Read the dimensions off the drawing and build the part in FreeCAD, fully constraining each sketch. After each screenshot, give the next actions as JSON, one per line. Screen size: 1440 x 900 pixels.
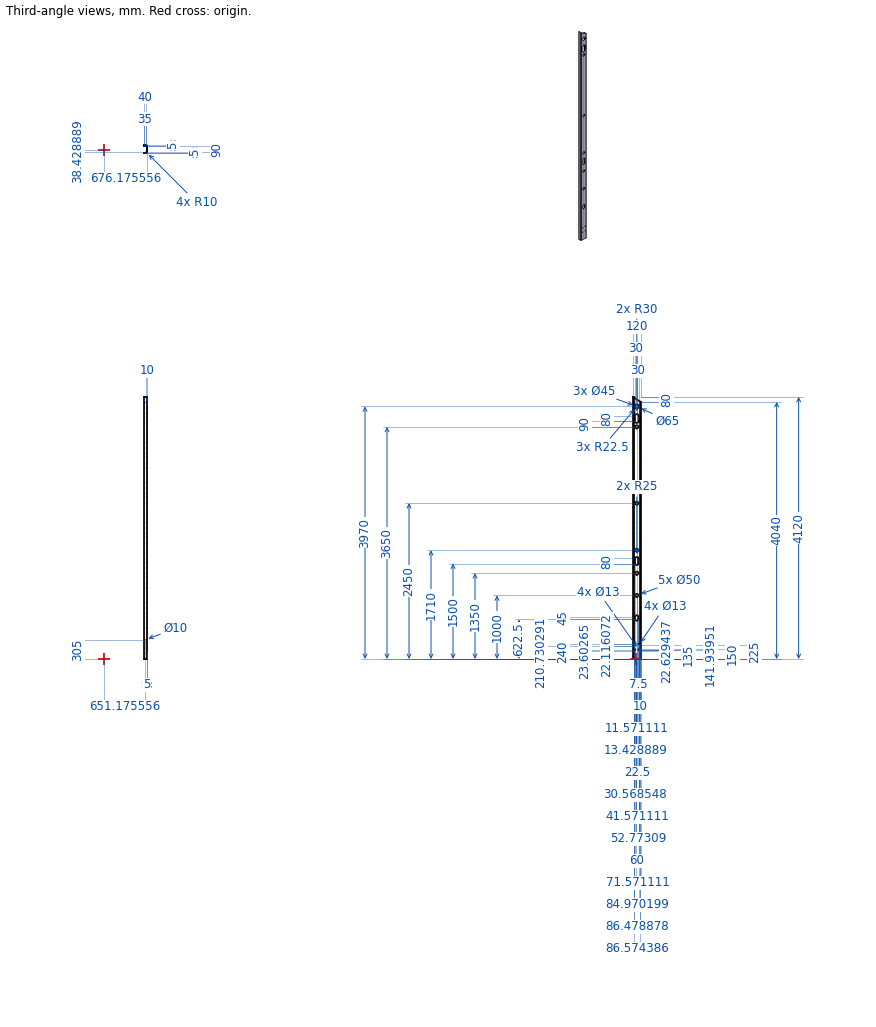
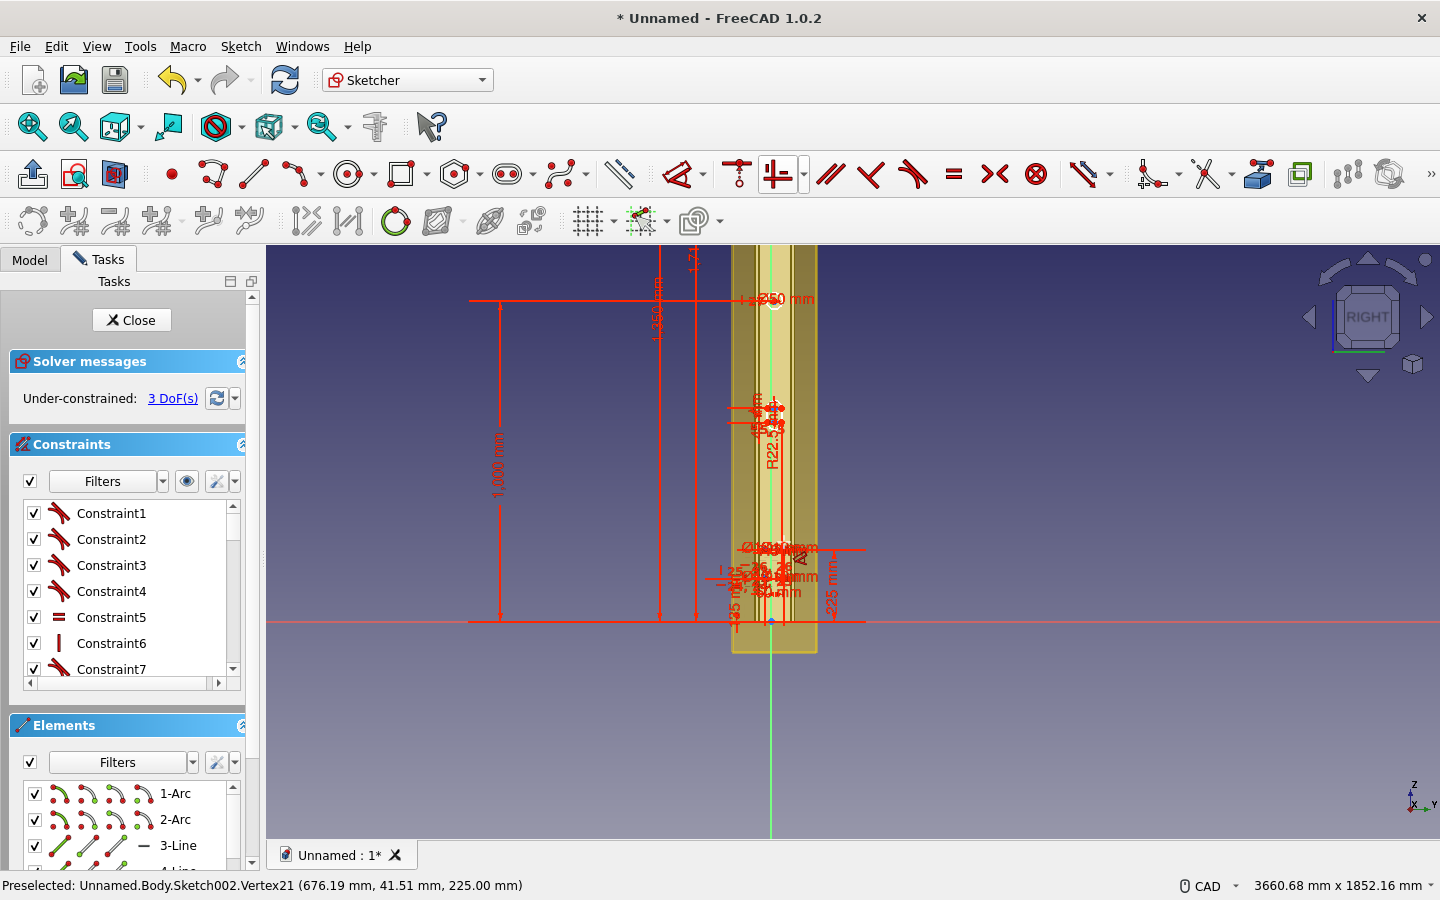
{"action": "scroll", "coordinate": [789, 784], "scroll_direction": "down", "scroll_amount": 6}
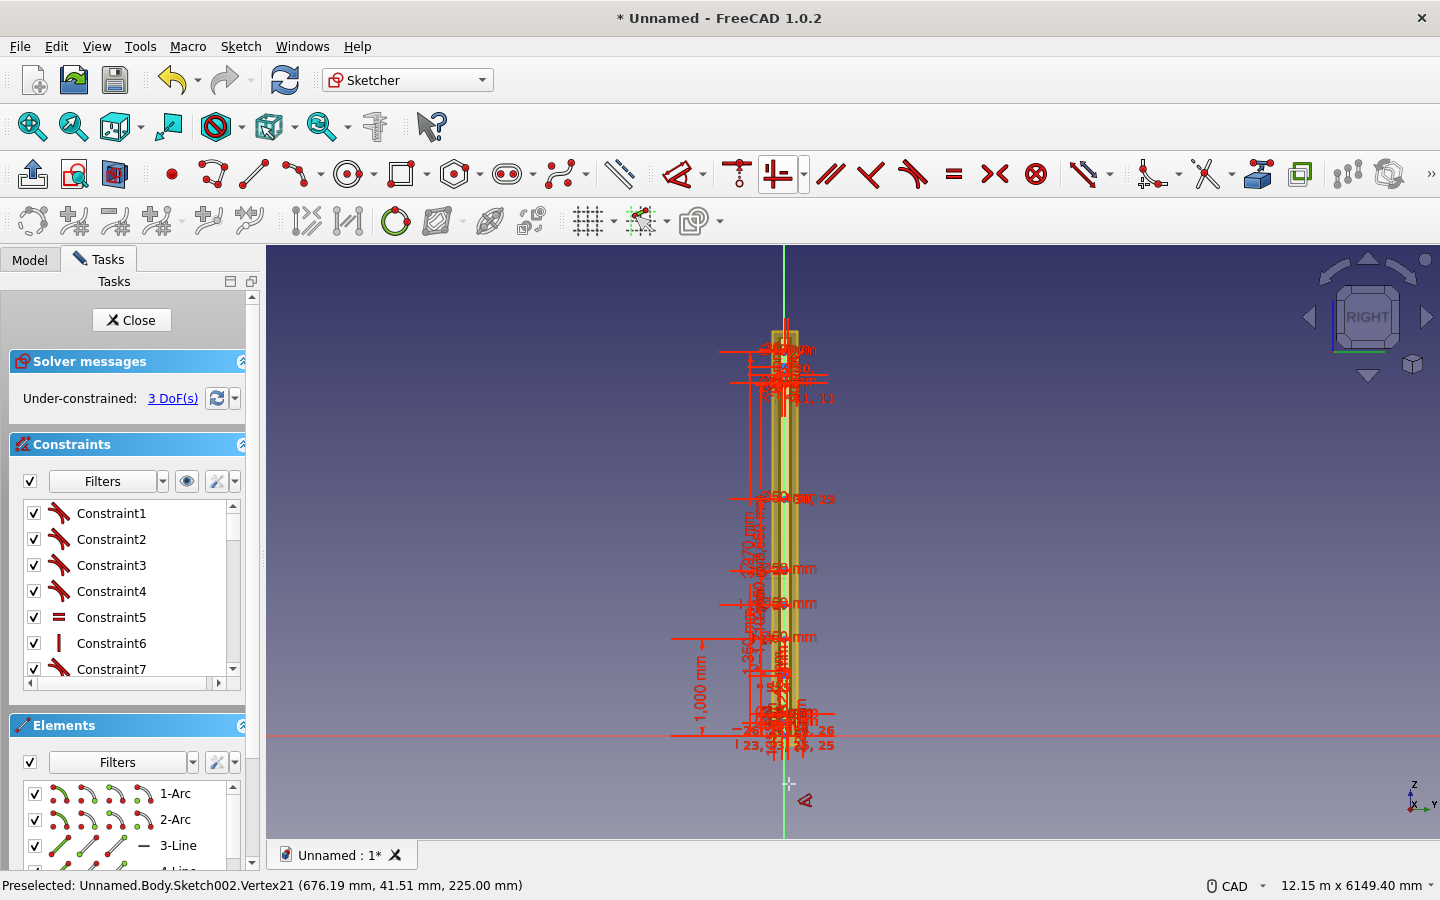
{"action": "scroll", "coordinate": [787, 671], "scroll_direction": "up", "scroll_amount": 15}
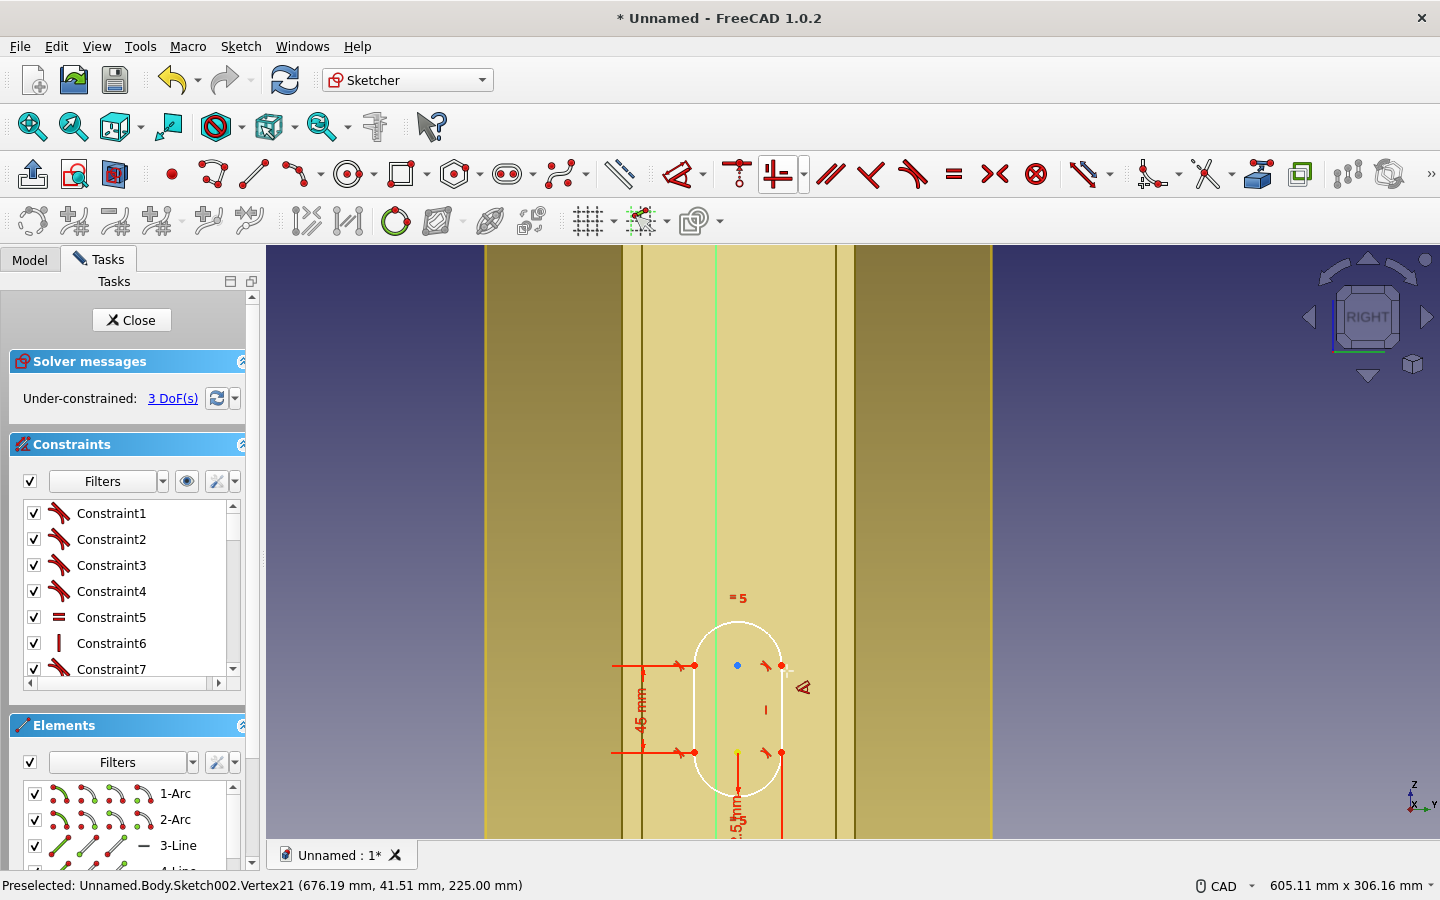
{"action": "left_click", "coordinate": [782, 666]}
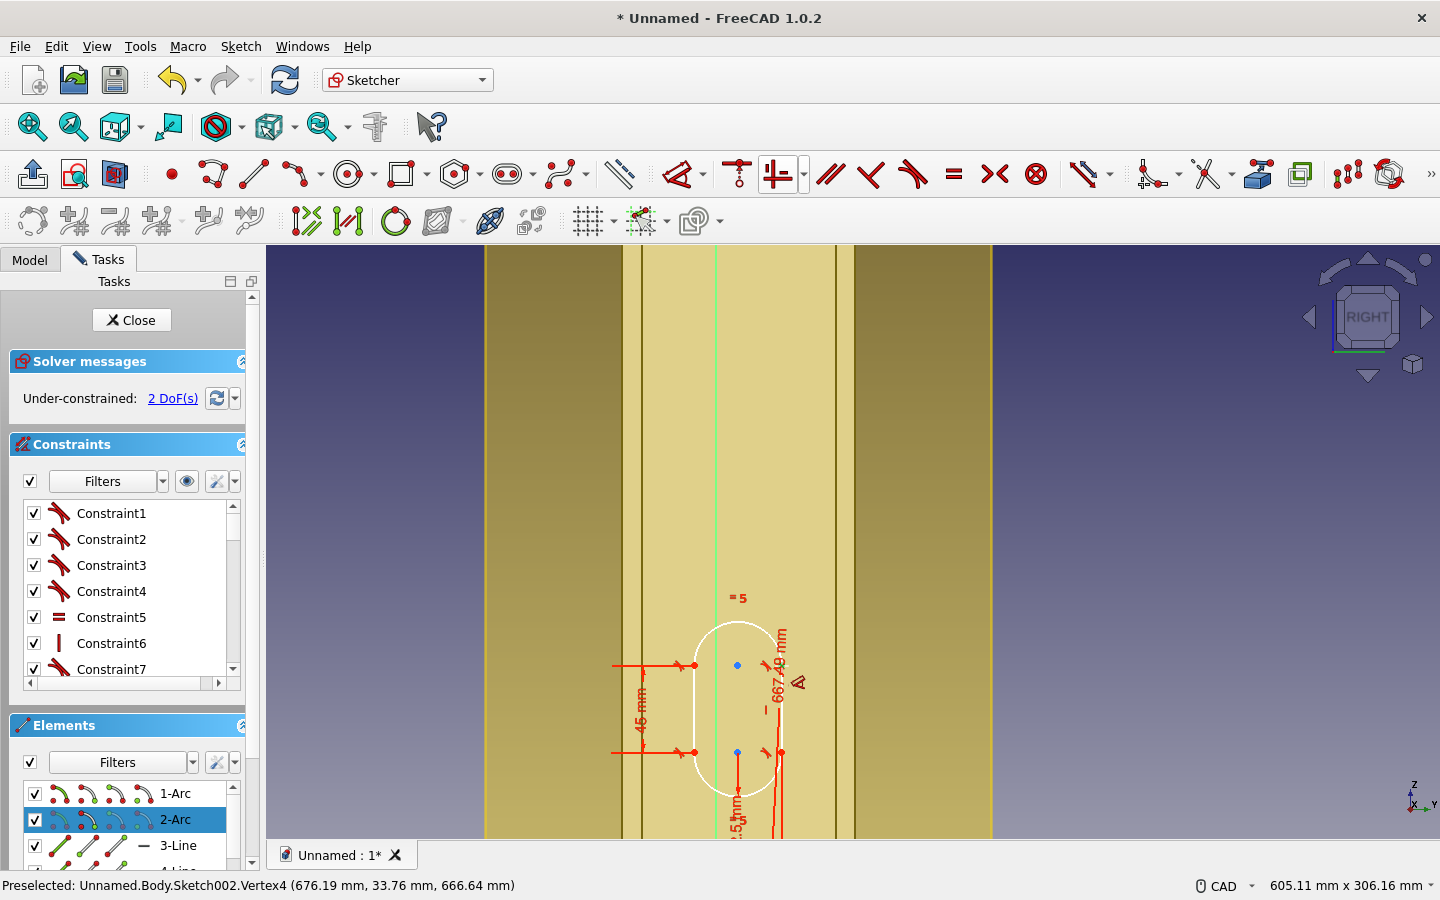
{"action": "scroll", "coordinate": [787, 671], "scroll_direction": "down", "scroll_amount": 15}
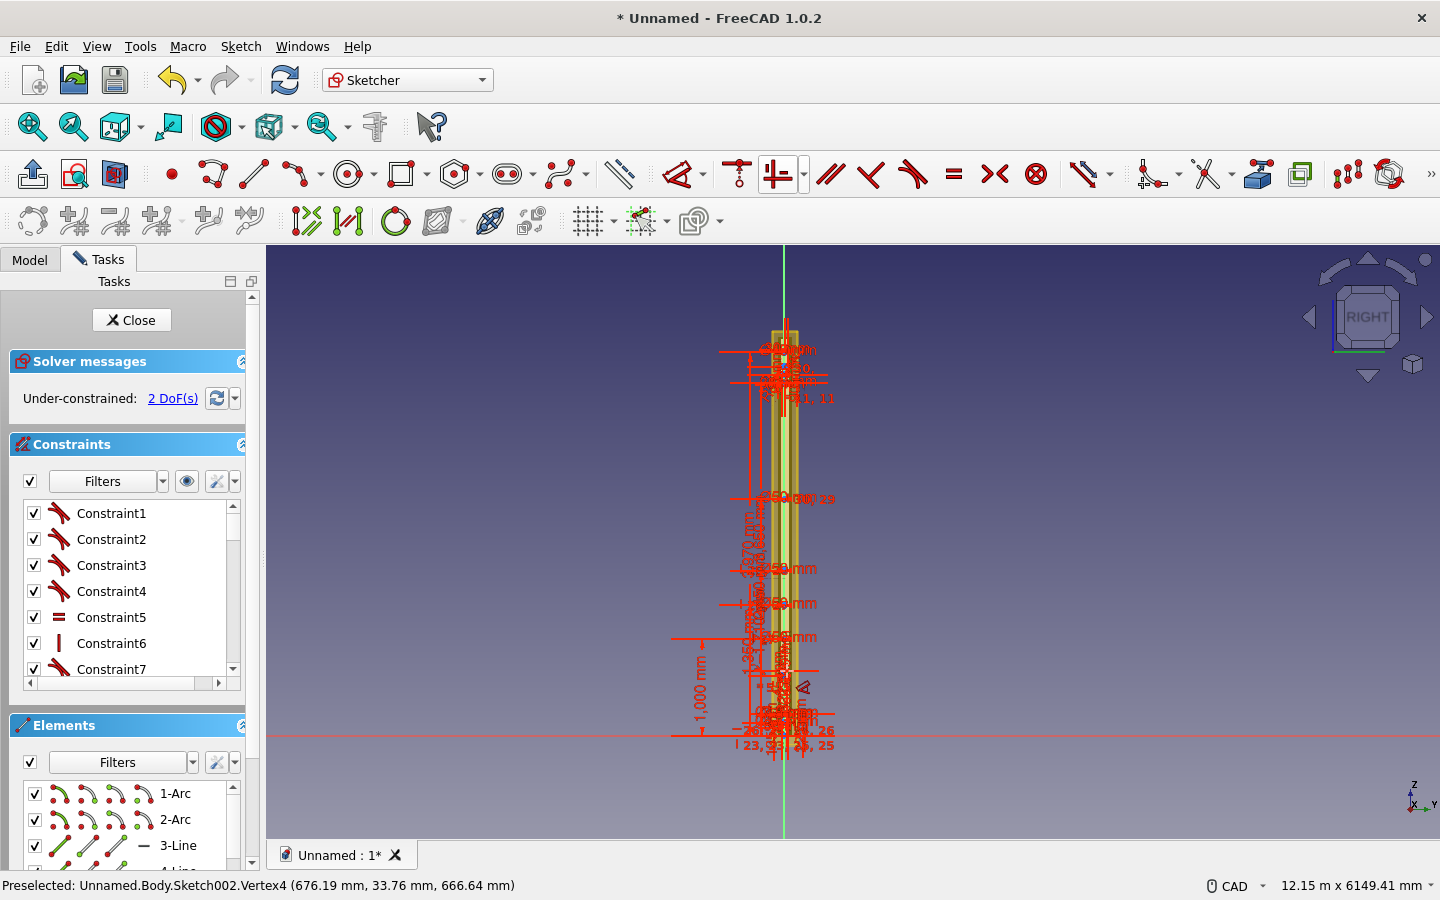
{"action": "scroll", "coordinate": [785, 639], "scroll_direction": "up", "scroll_amount": 15}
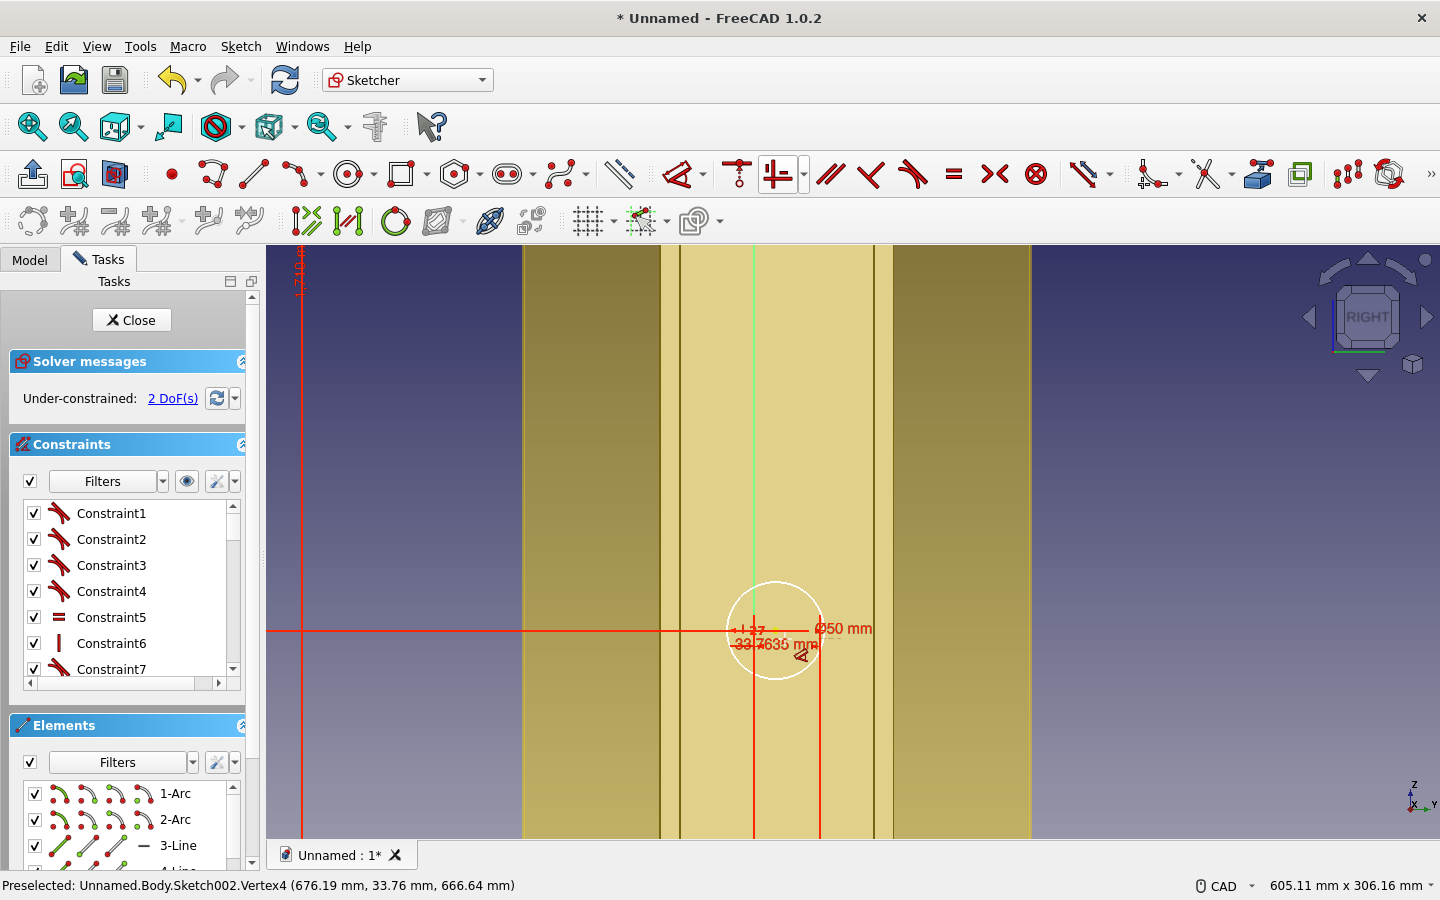
{"action": "left_click", "coordinate": [776, 631]}
{"action": "left_click", "coordinate": [782, 597]}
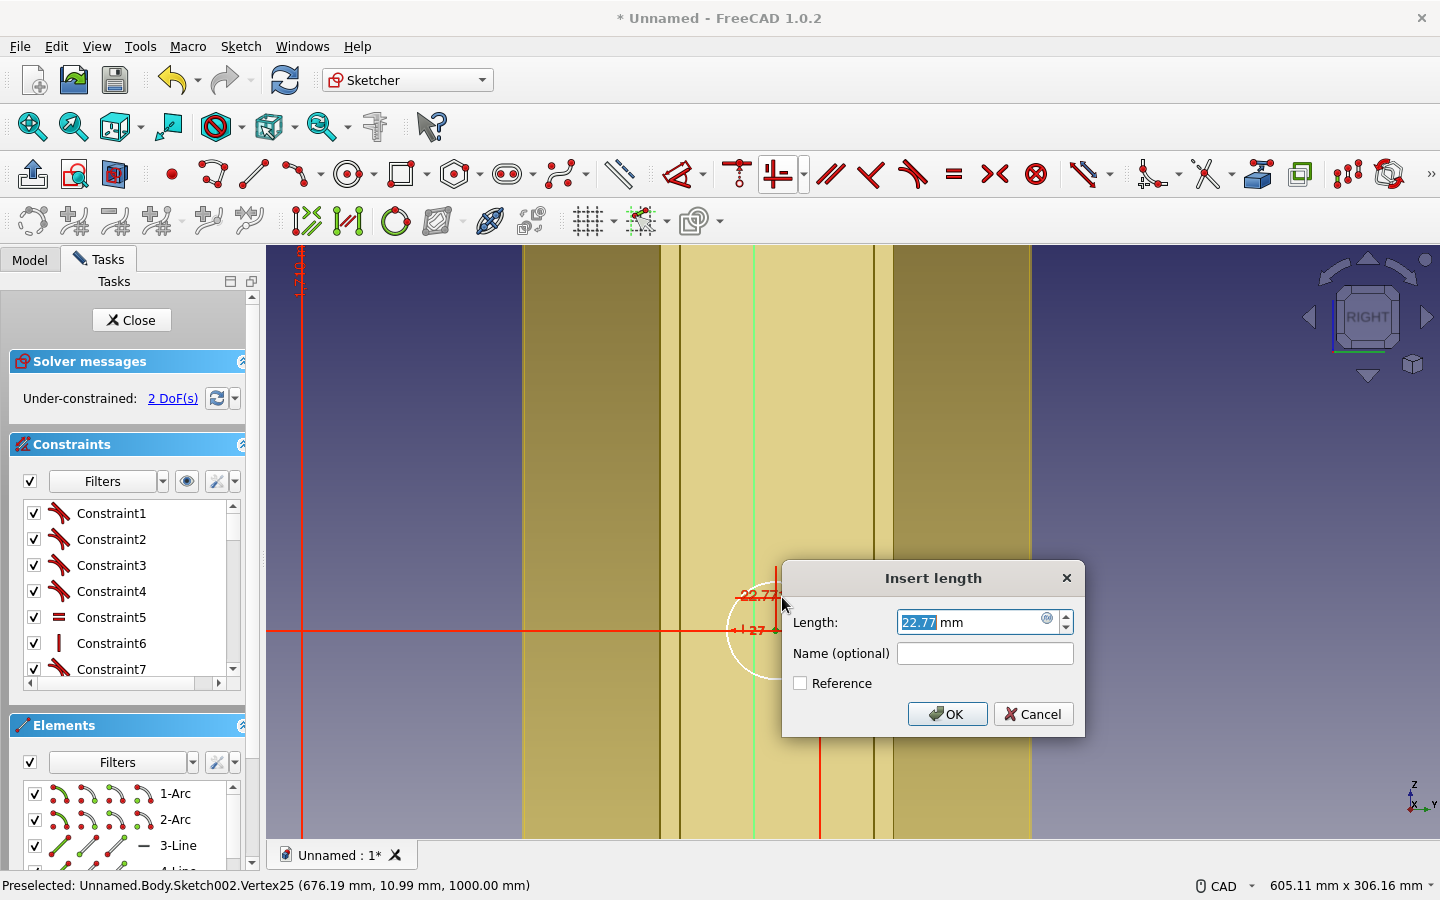
{"action": "type", "text": "22.5"}
{"action": "key", "text": "Return"}